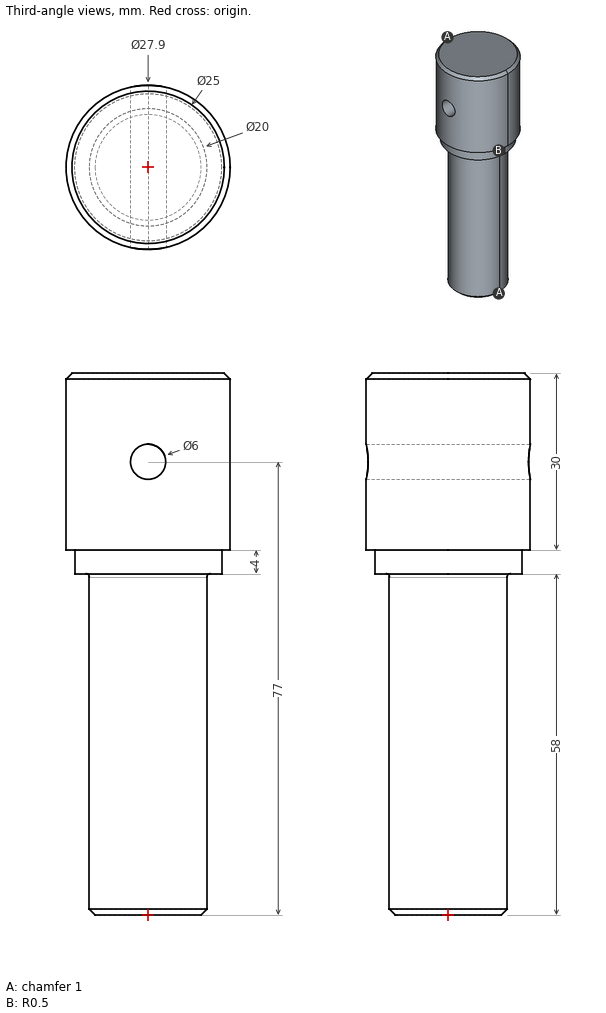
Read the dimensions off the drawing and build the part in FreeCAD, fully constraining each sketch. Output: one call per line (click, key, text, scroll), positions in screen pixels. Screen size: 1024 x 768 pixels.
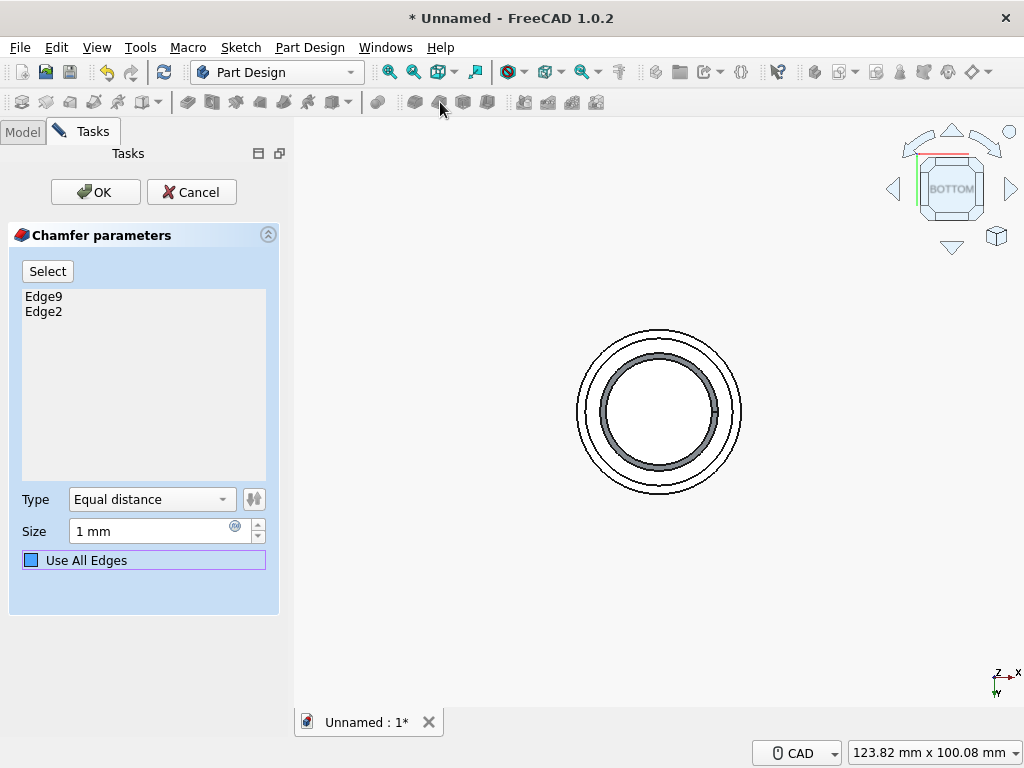
click(96, 192)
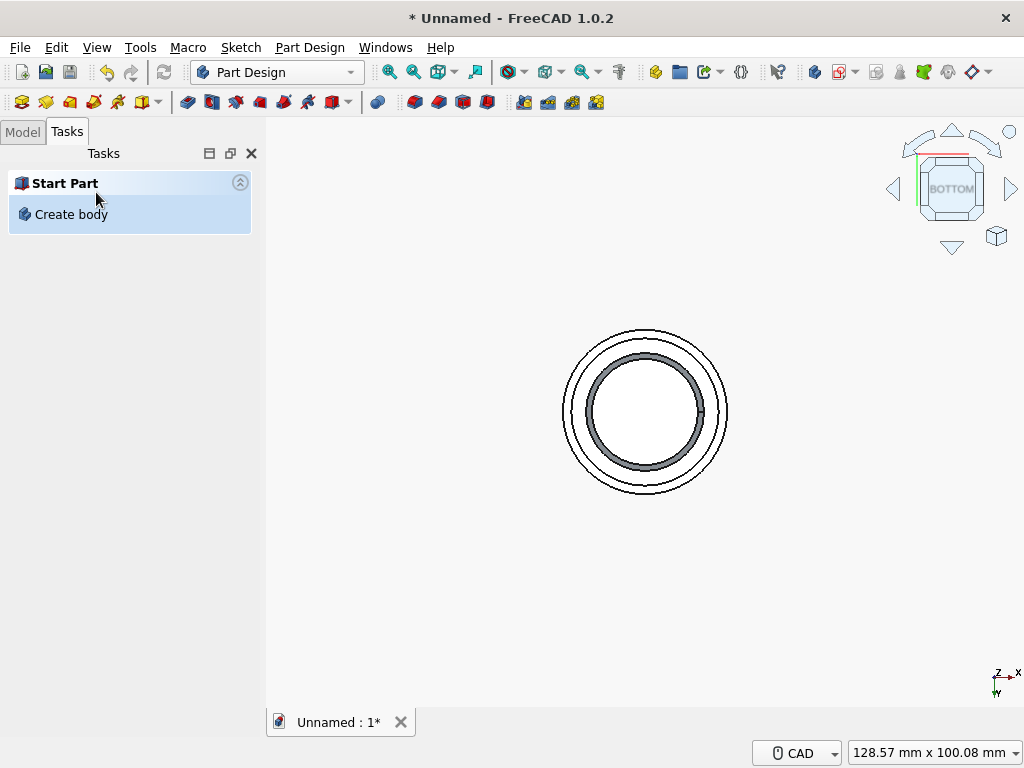
click(390, 72)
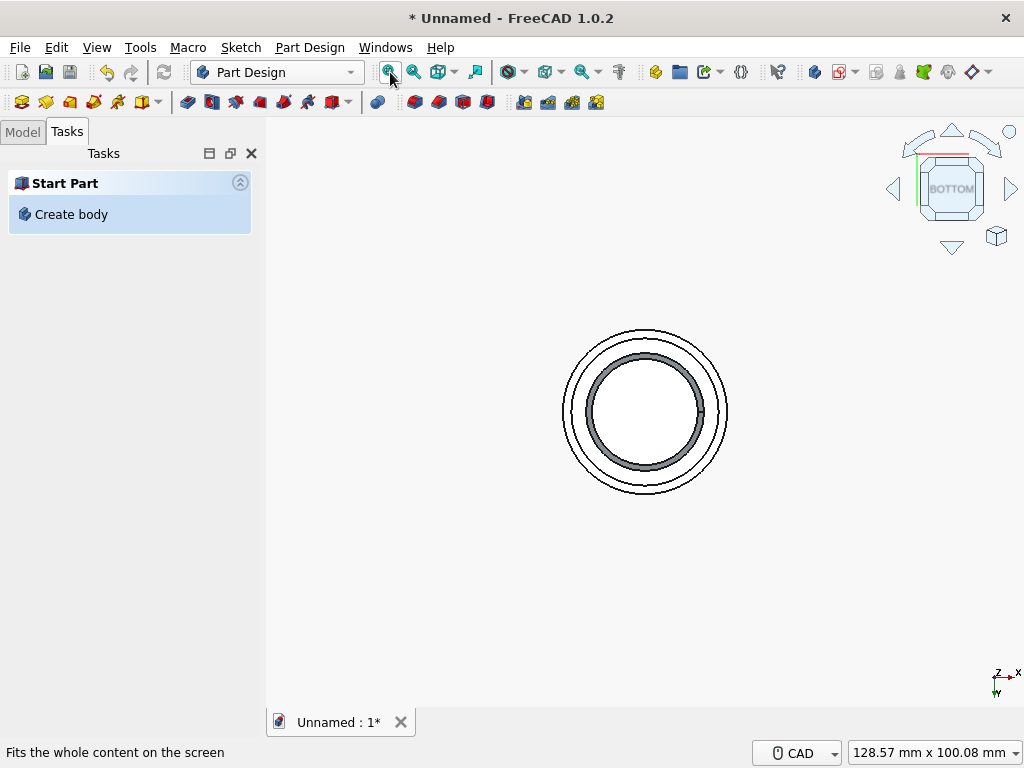
key(0)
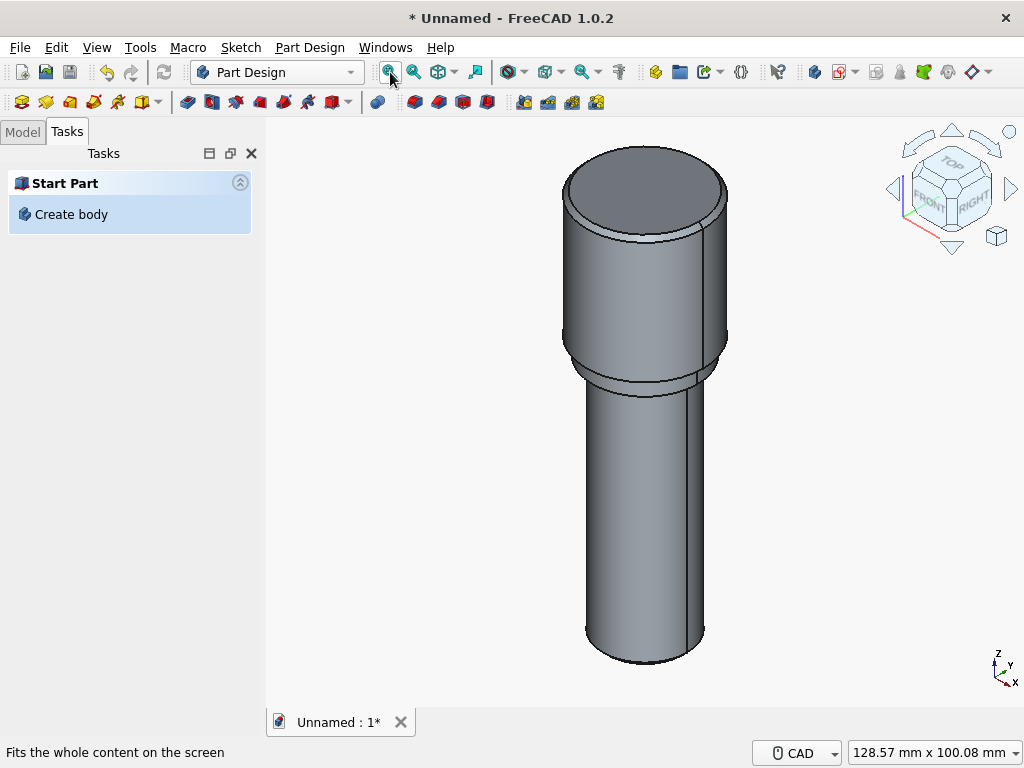
key(2)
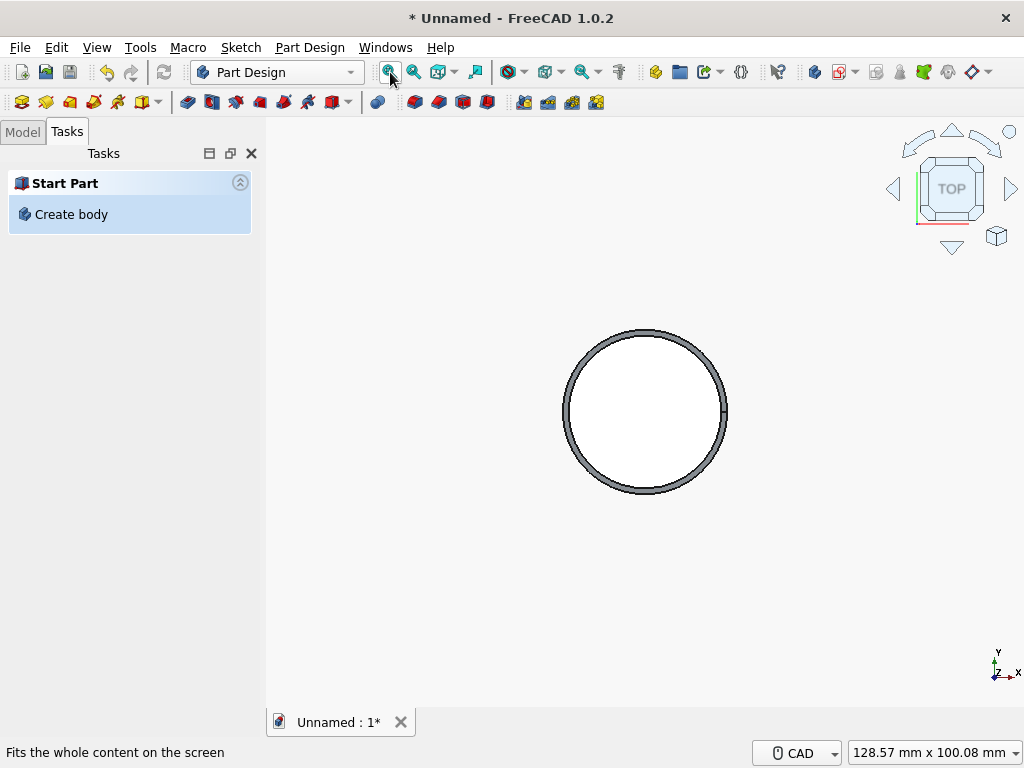
click(390, 72)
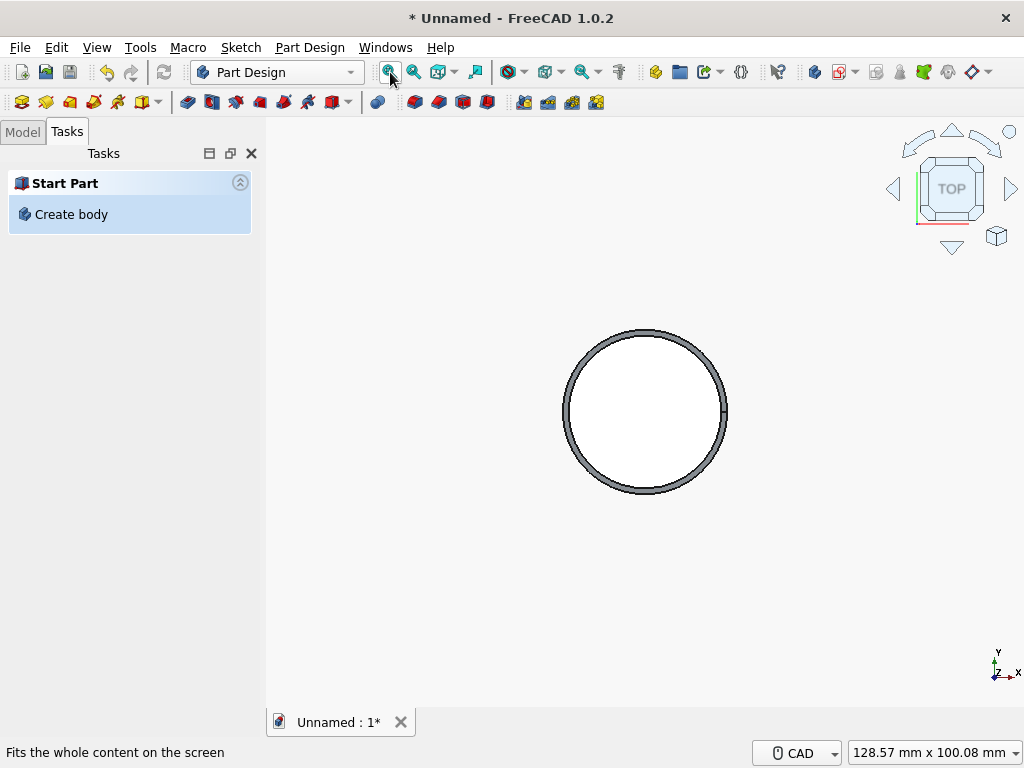
key(1)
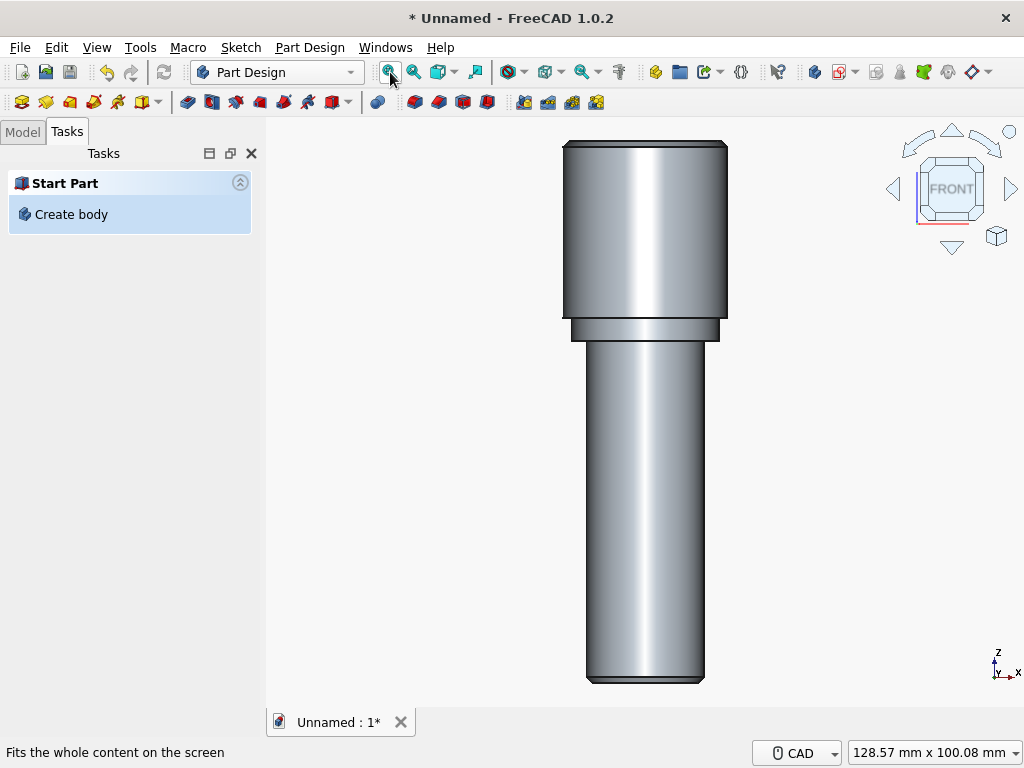
key(3)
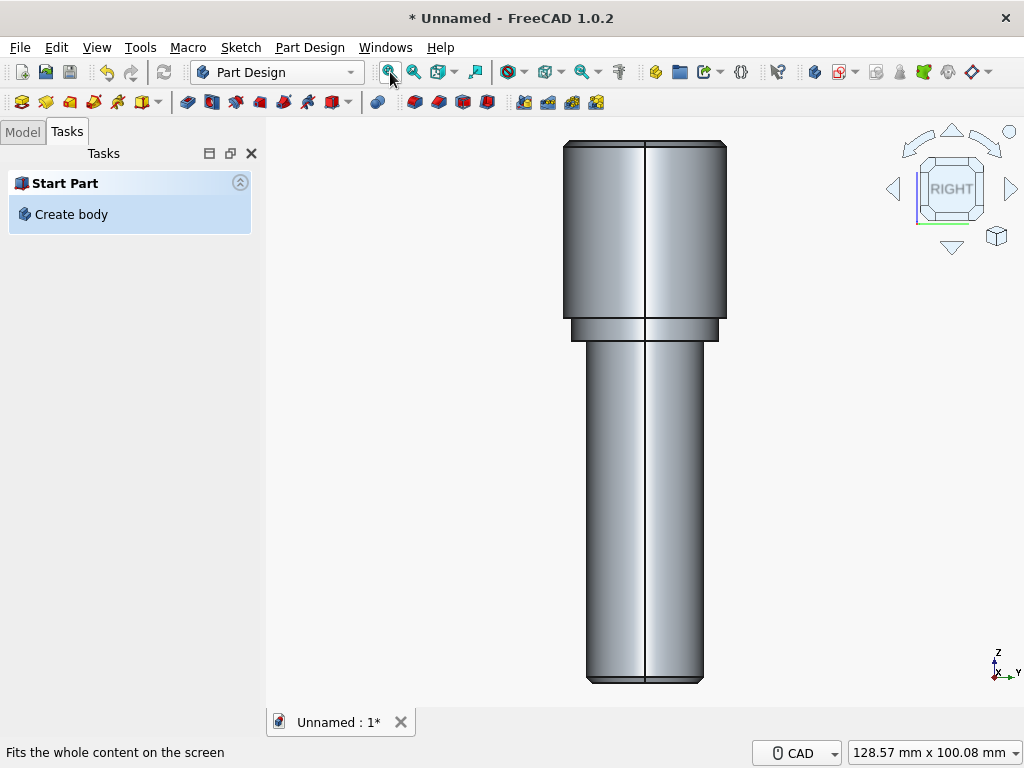
key(5)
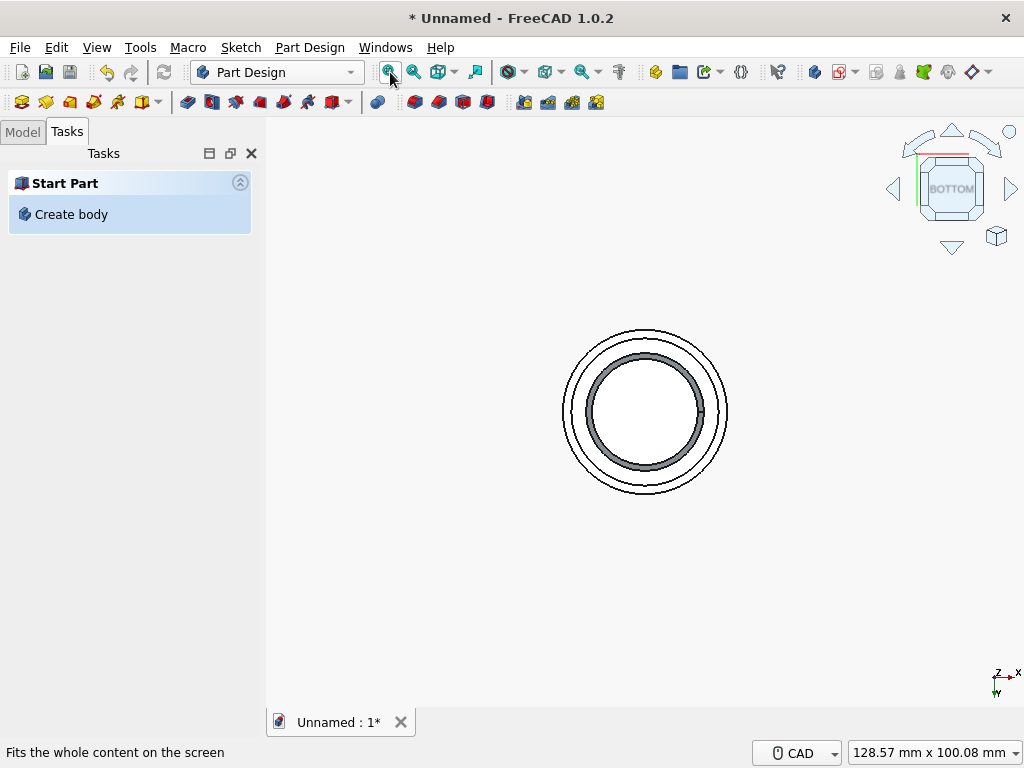
click(390, 72)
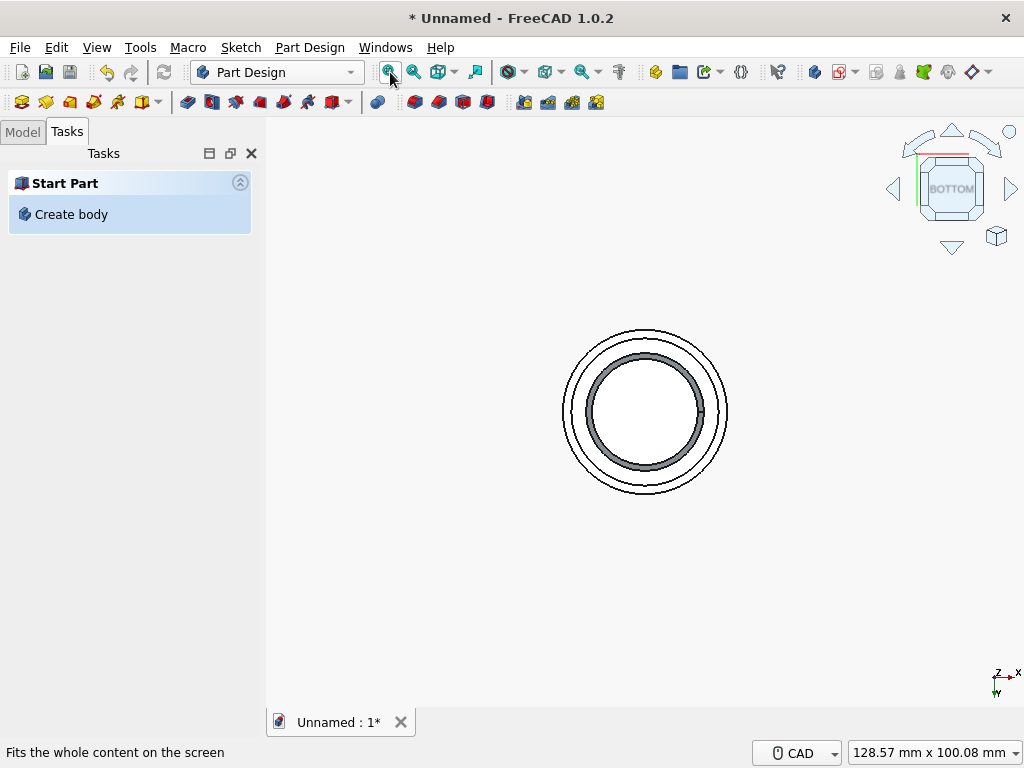
key(4)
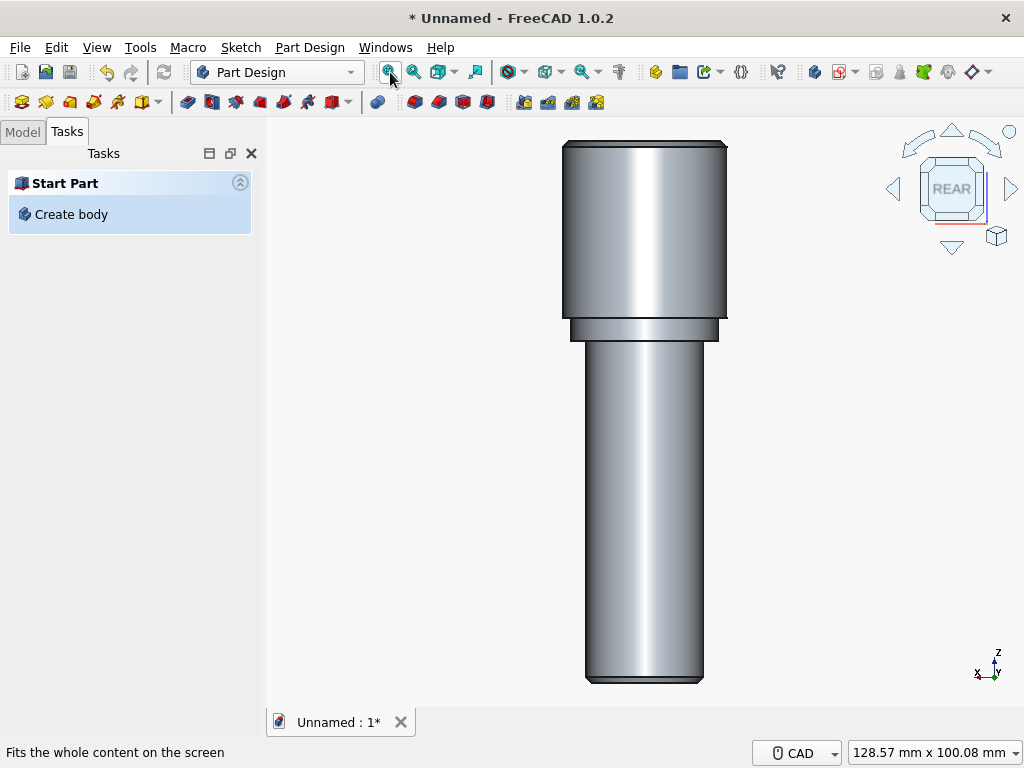
key(6)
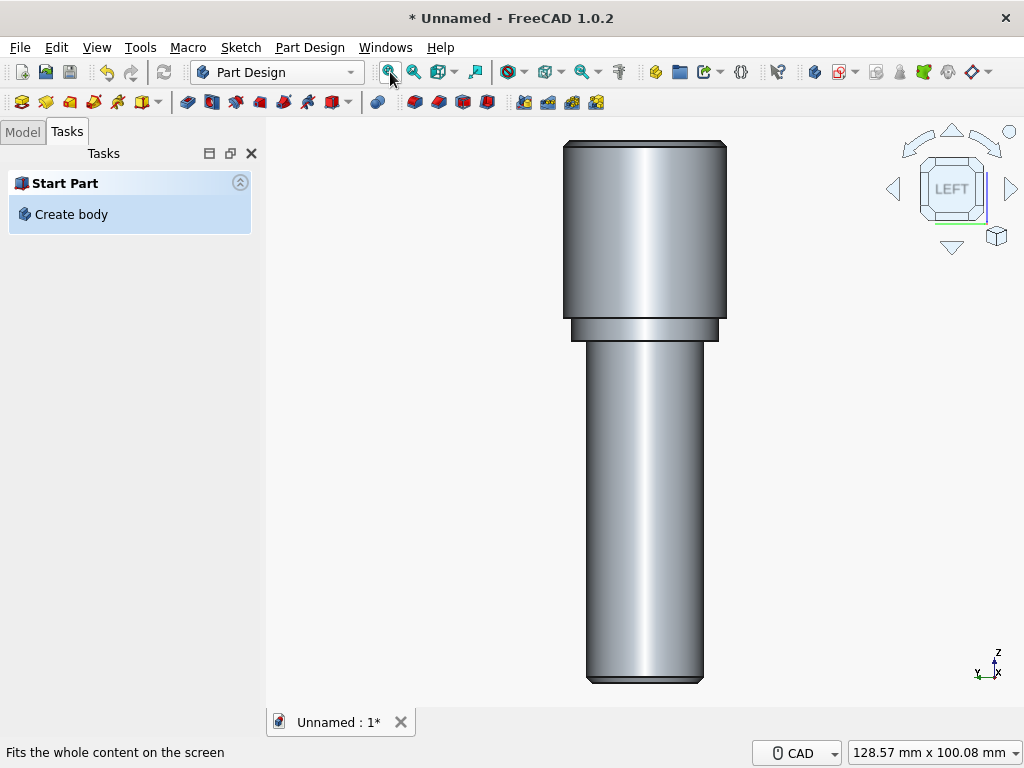
key(v)
key(3)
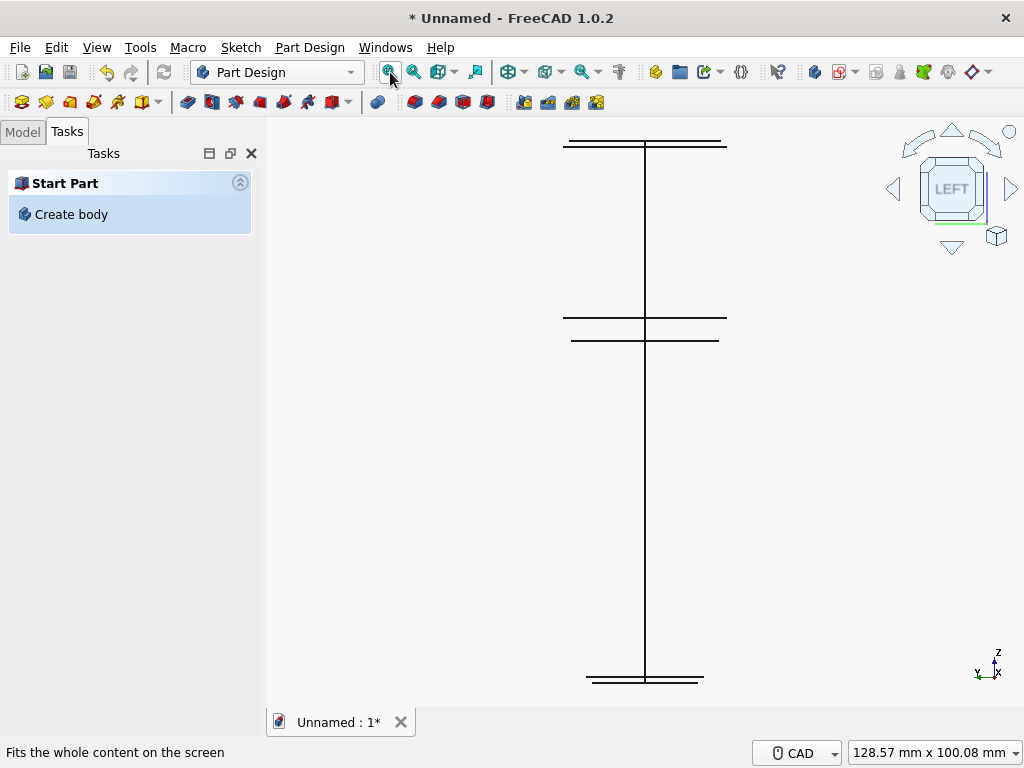
key(0)